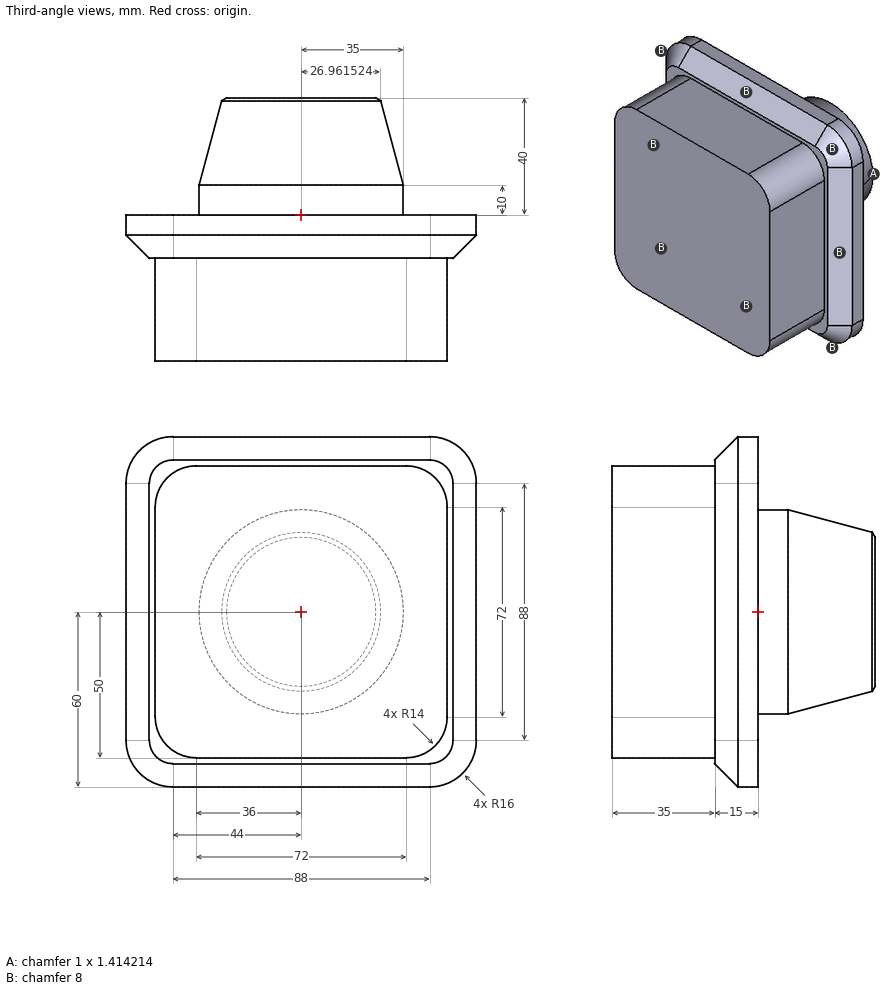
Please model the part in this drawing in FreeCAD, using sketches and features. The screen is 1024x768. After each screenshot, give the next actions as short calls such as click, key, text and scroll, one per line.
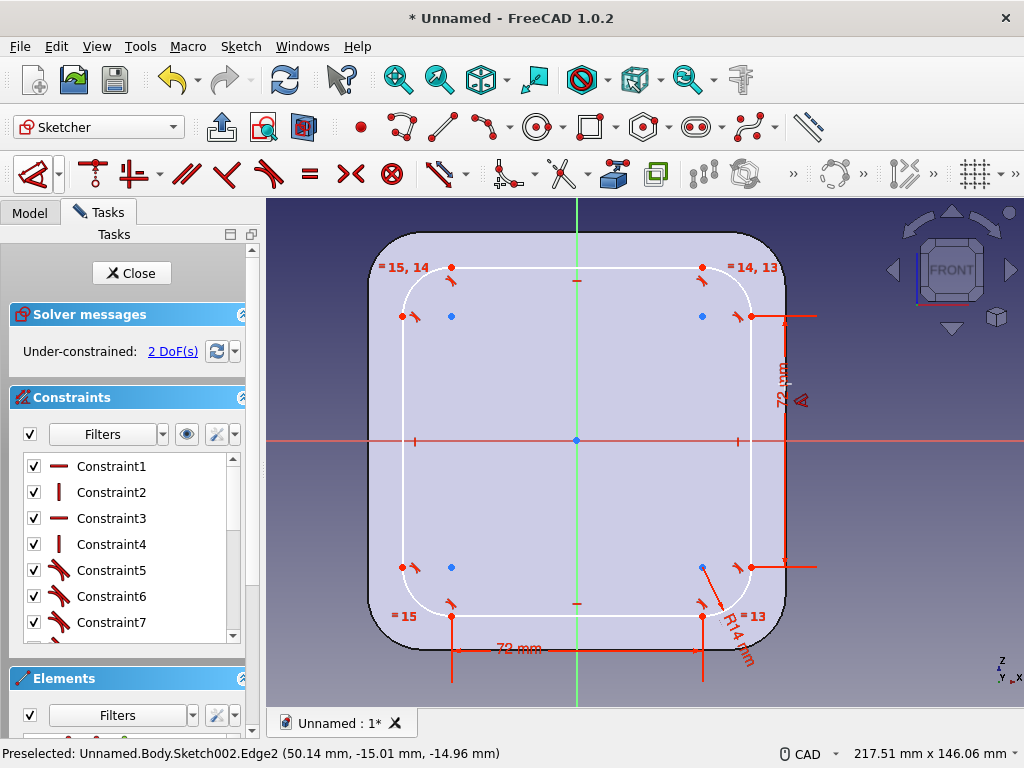
click(452, 616)
click(514, 407)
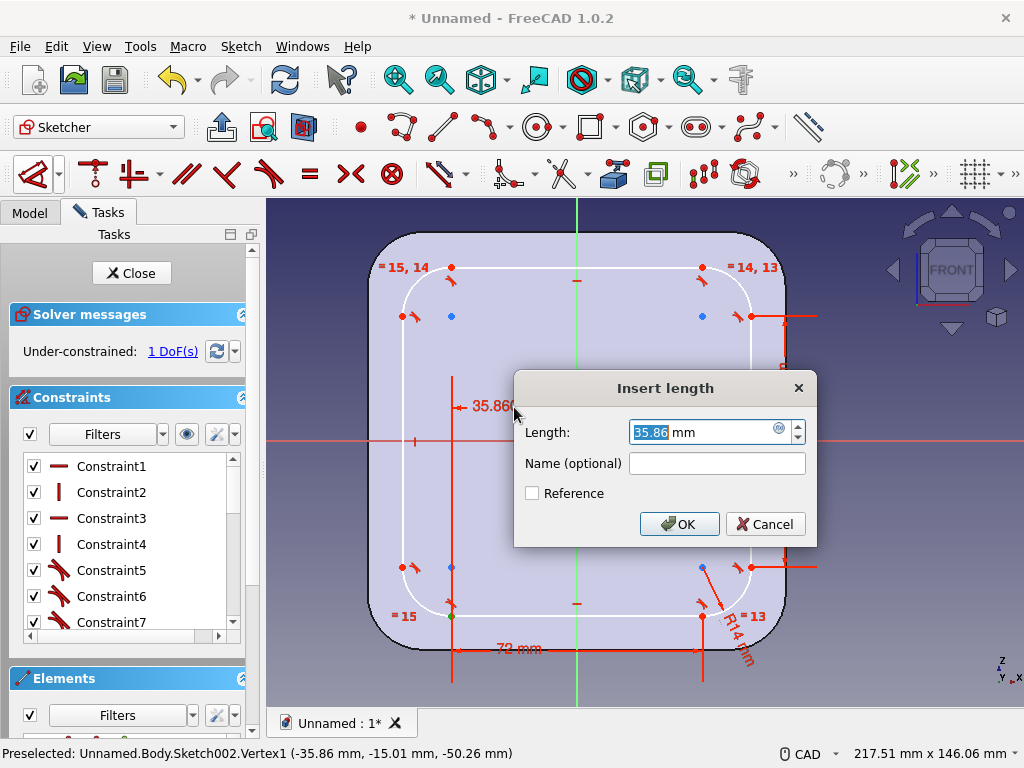
text(36)
key(Return)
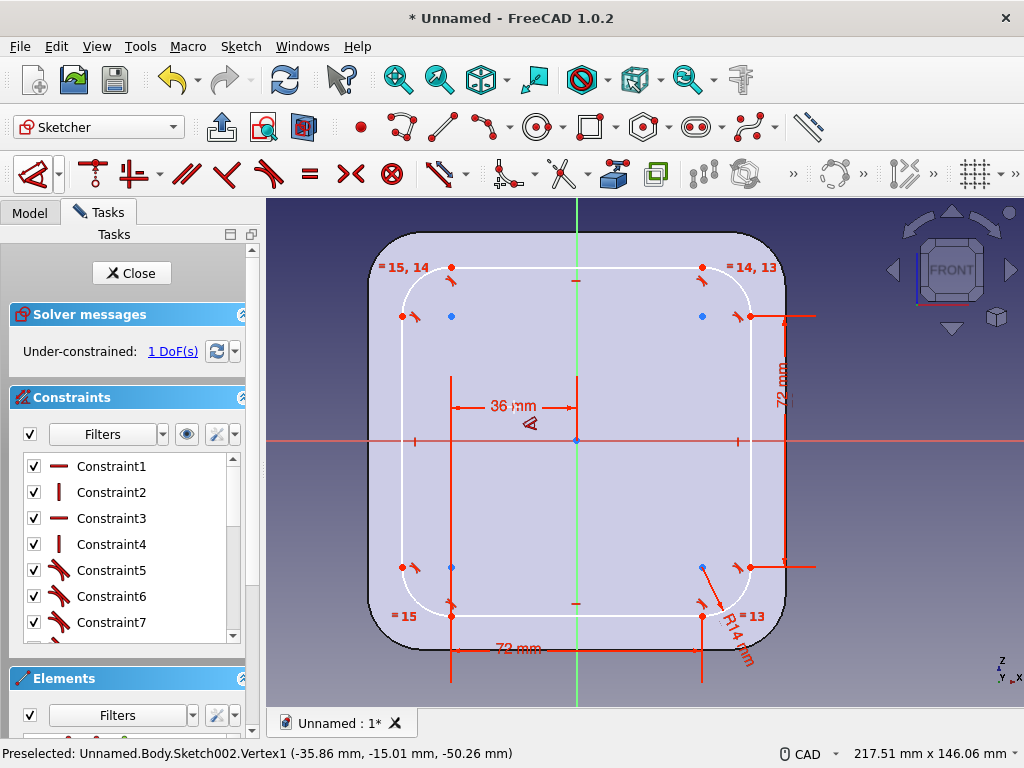
click(451, 616)
click(417, 528)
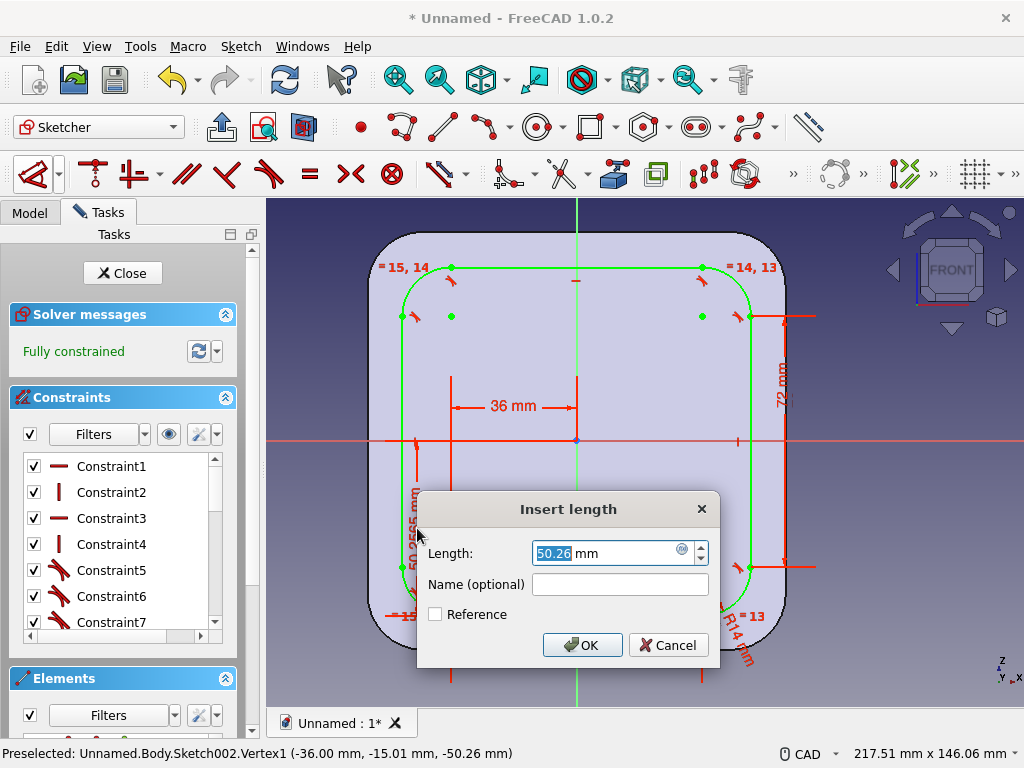
text(50)
key(Return)
key(Escape)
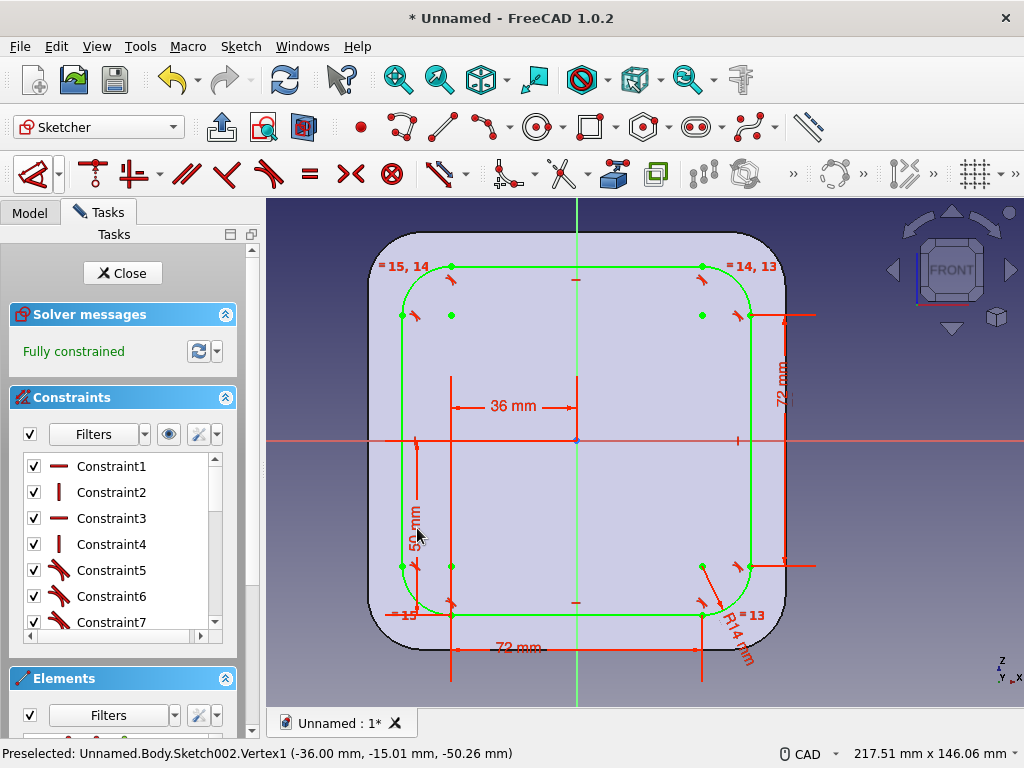
click(123, 273)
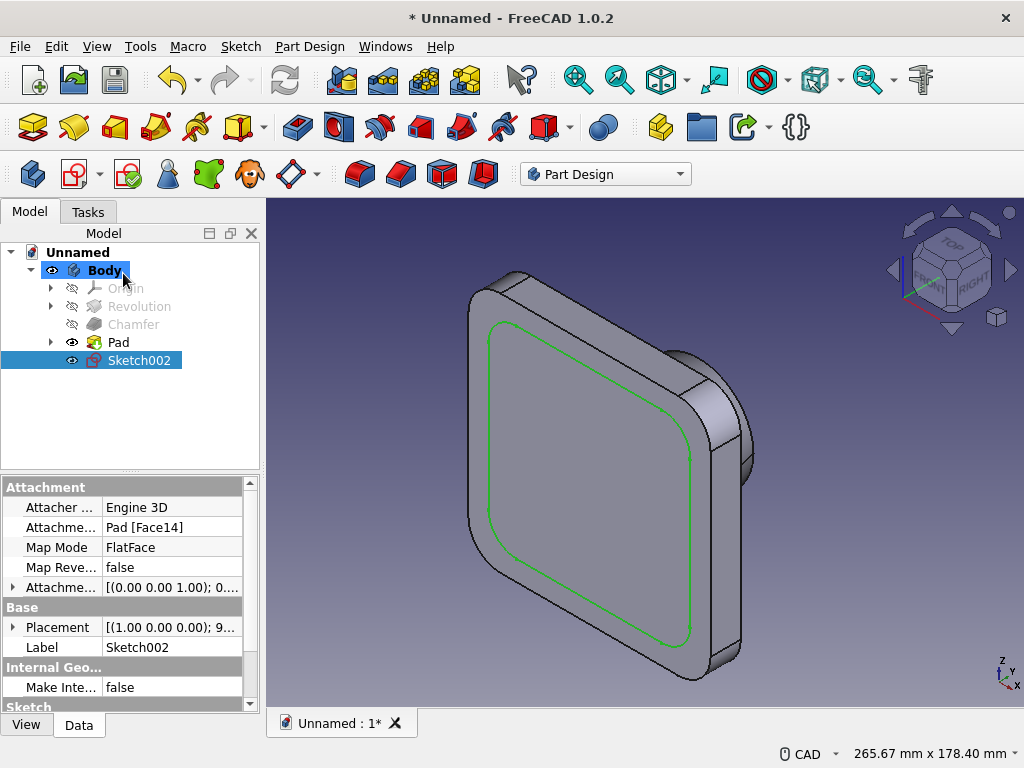
click(33, 128)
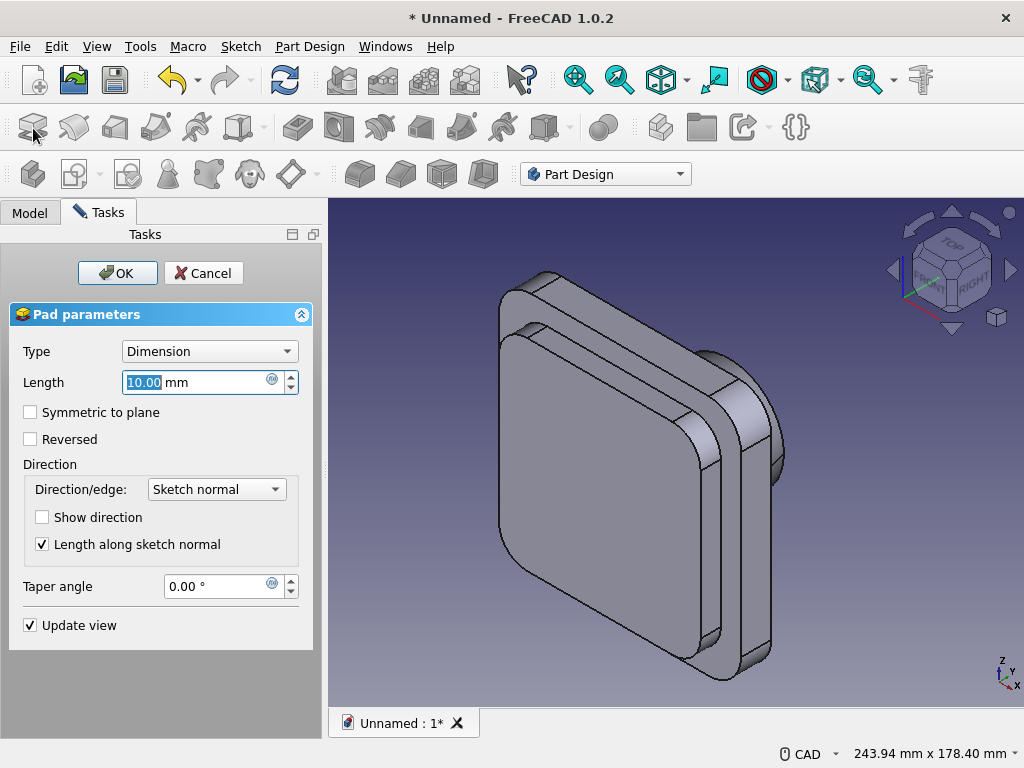
text(35)
key(Tab)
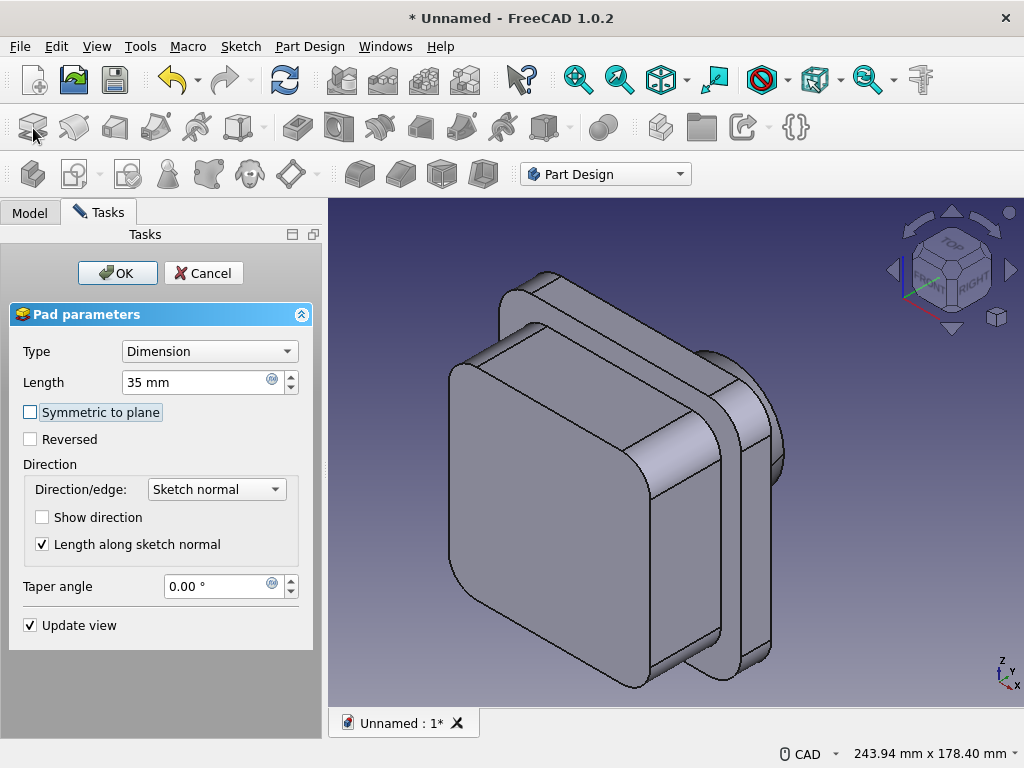
click(118, 273)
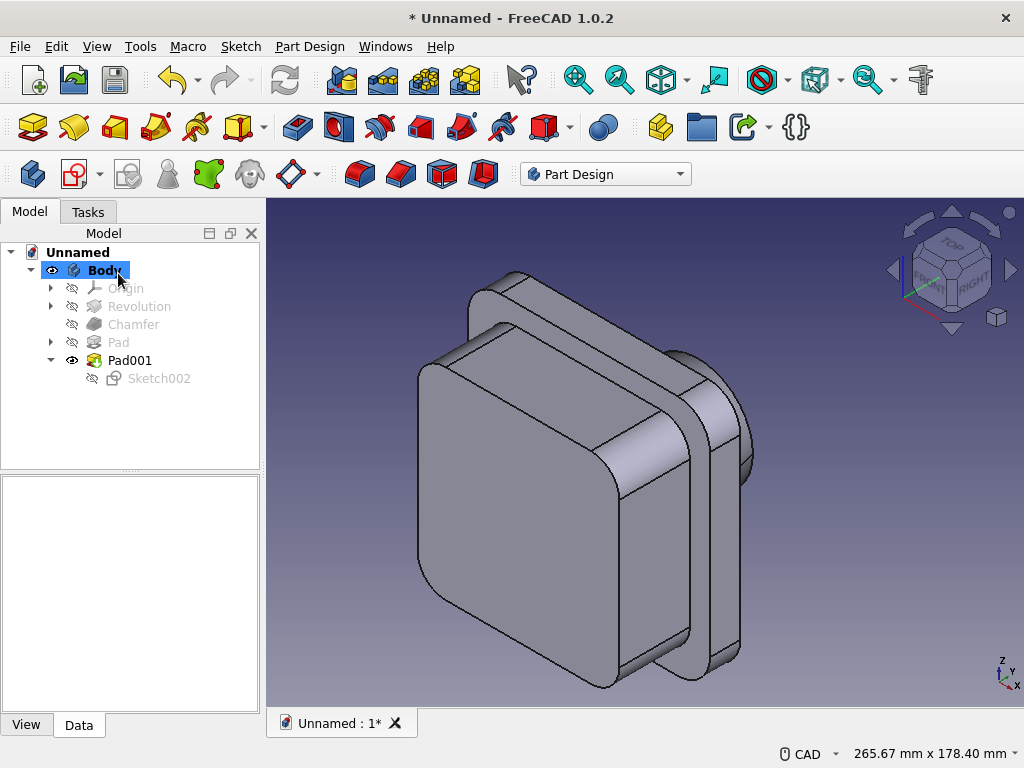
click(579, 80)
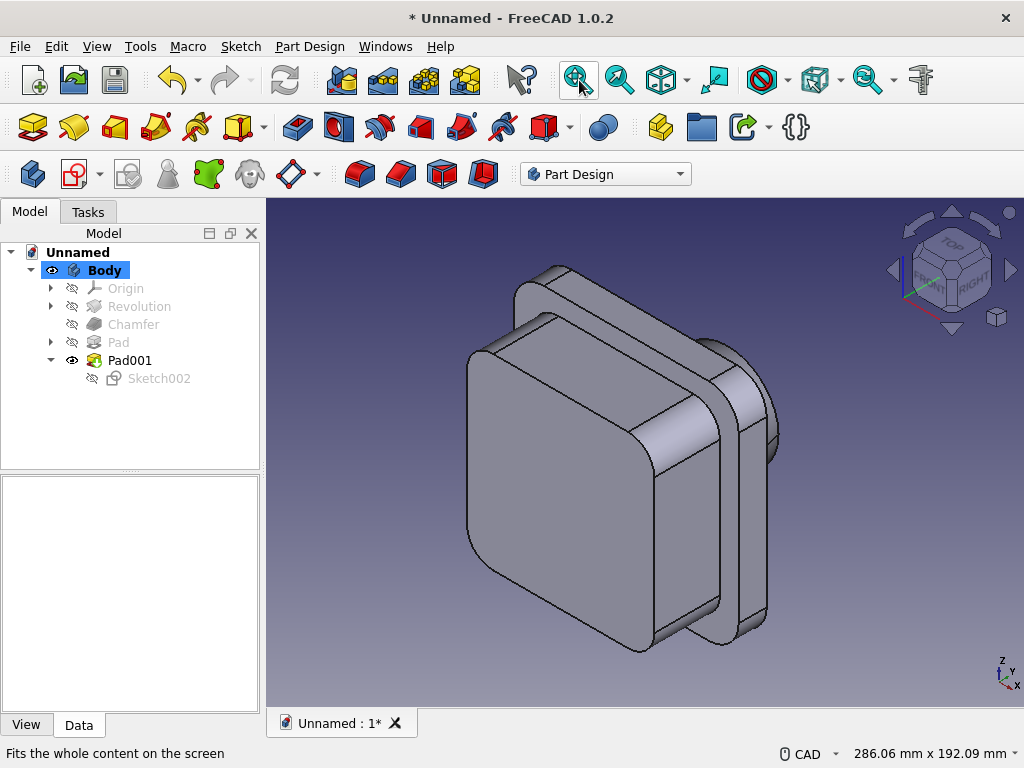
click(730, 642)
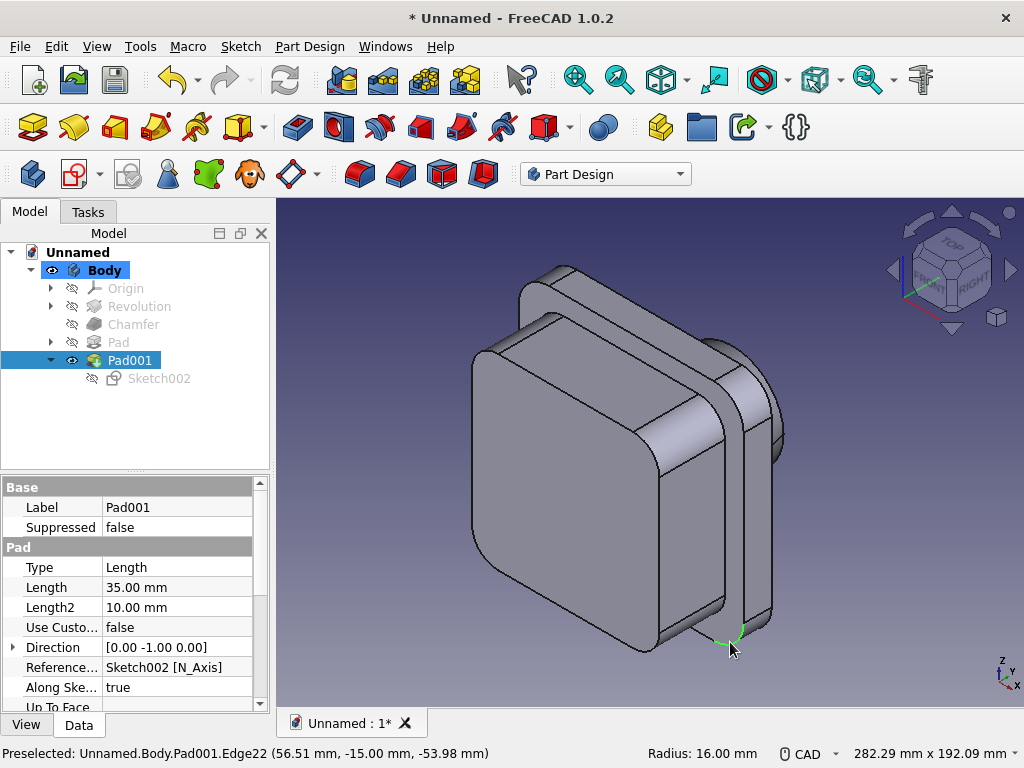
click(744, 527, ctrl)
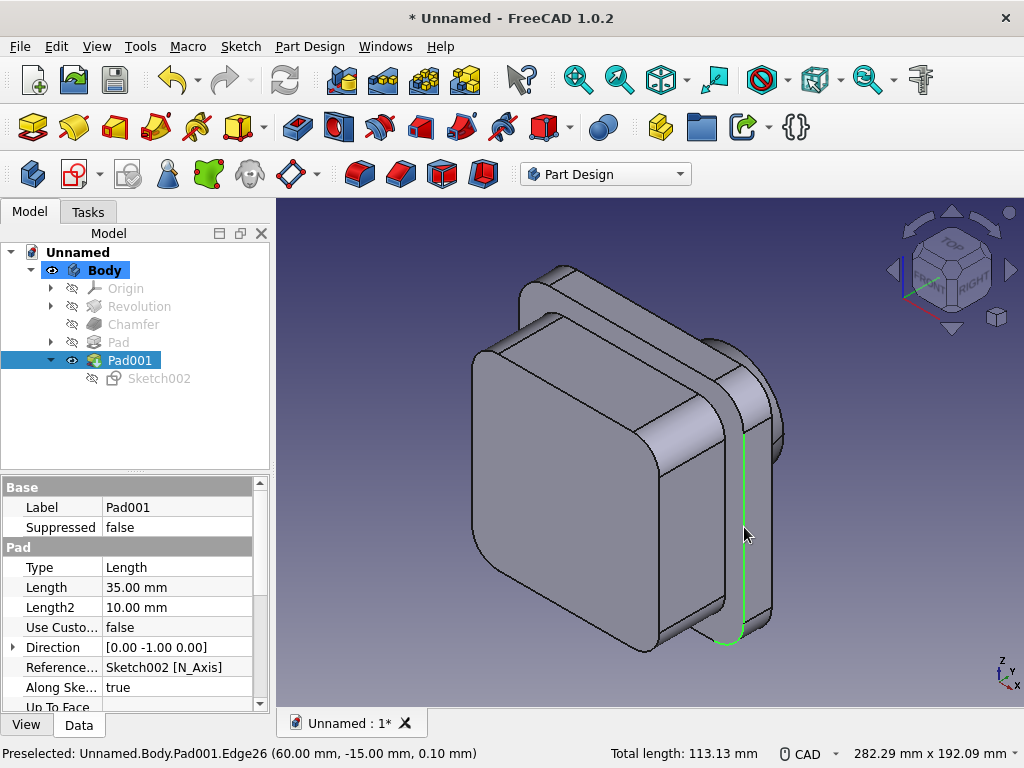
click(735, 402, ctrl)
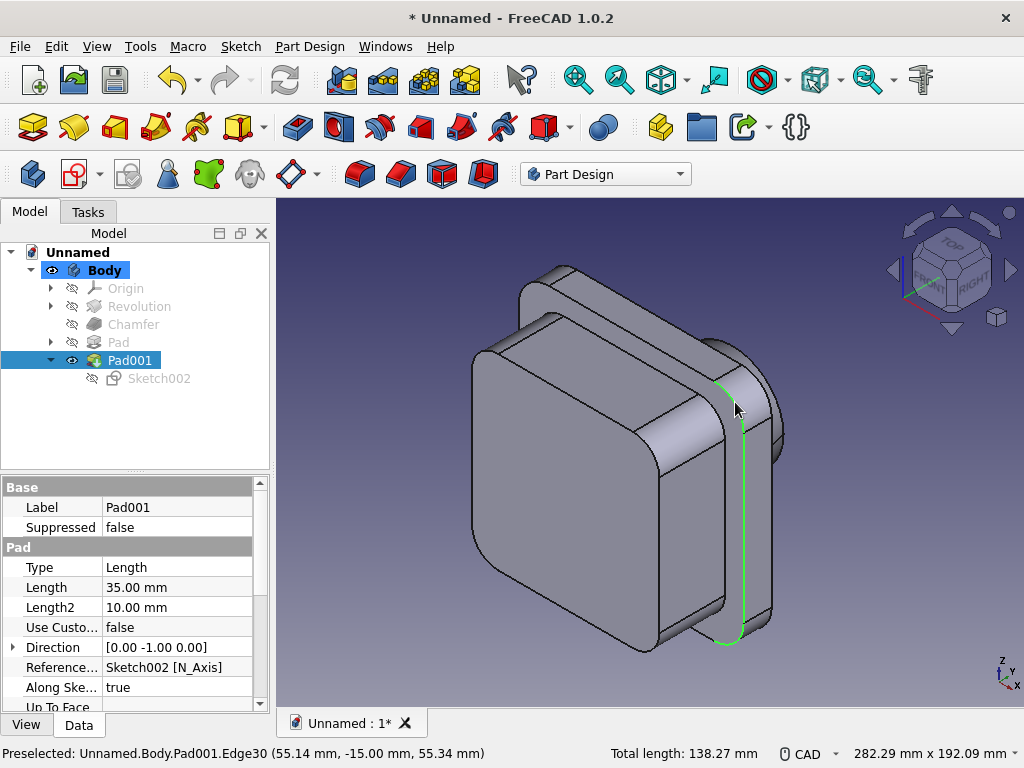
click(631, 333, ctrl)